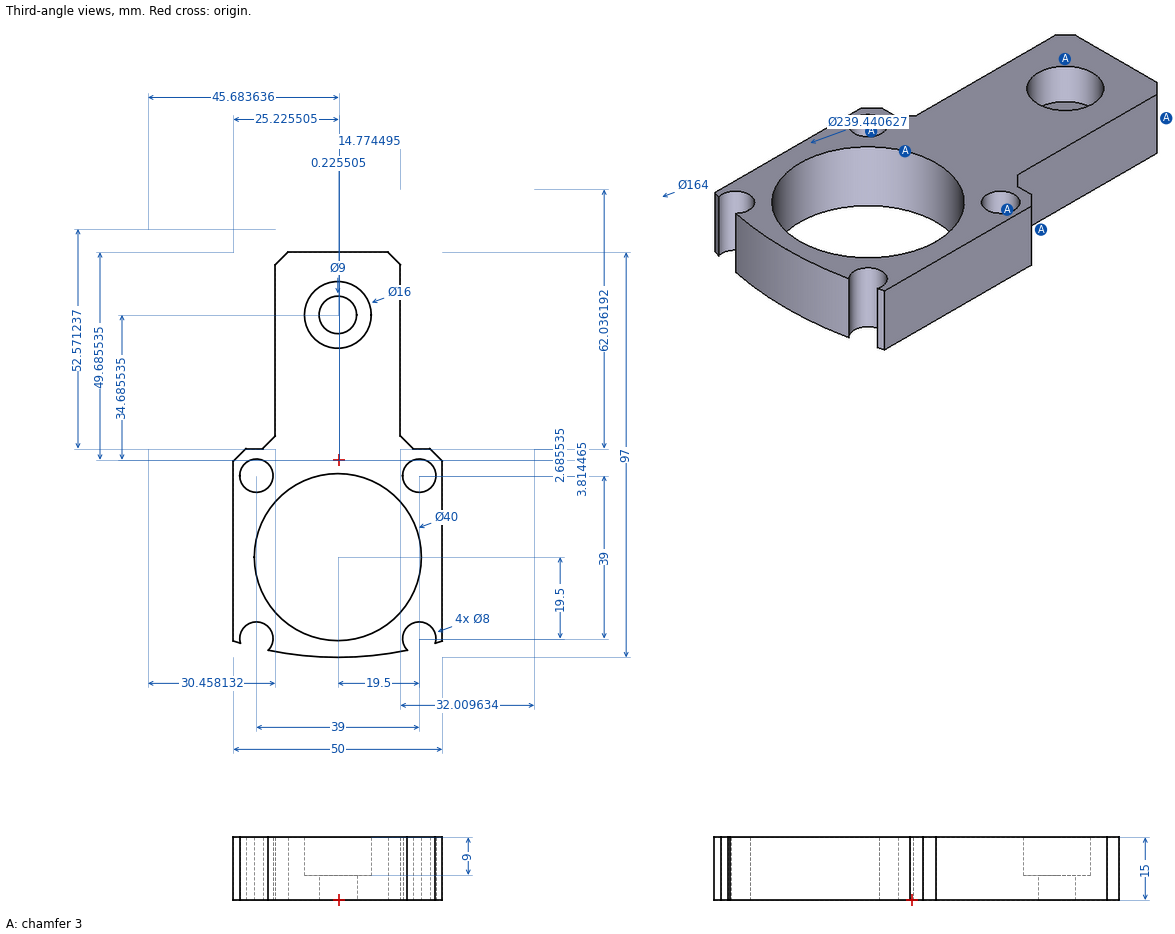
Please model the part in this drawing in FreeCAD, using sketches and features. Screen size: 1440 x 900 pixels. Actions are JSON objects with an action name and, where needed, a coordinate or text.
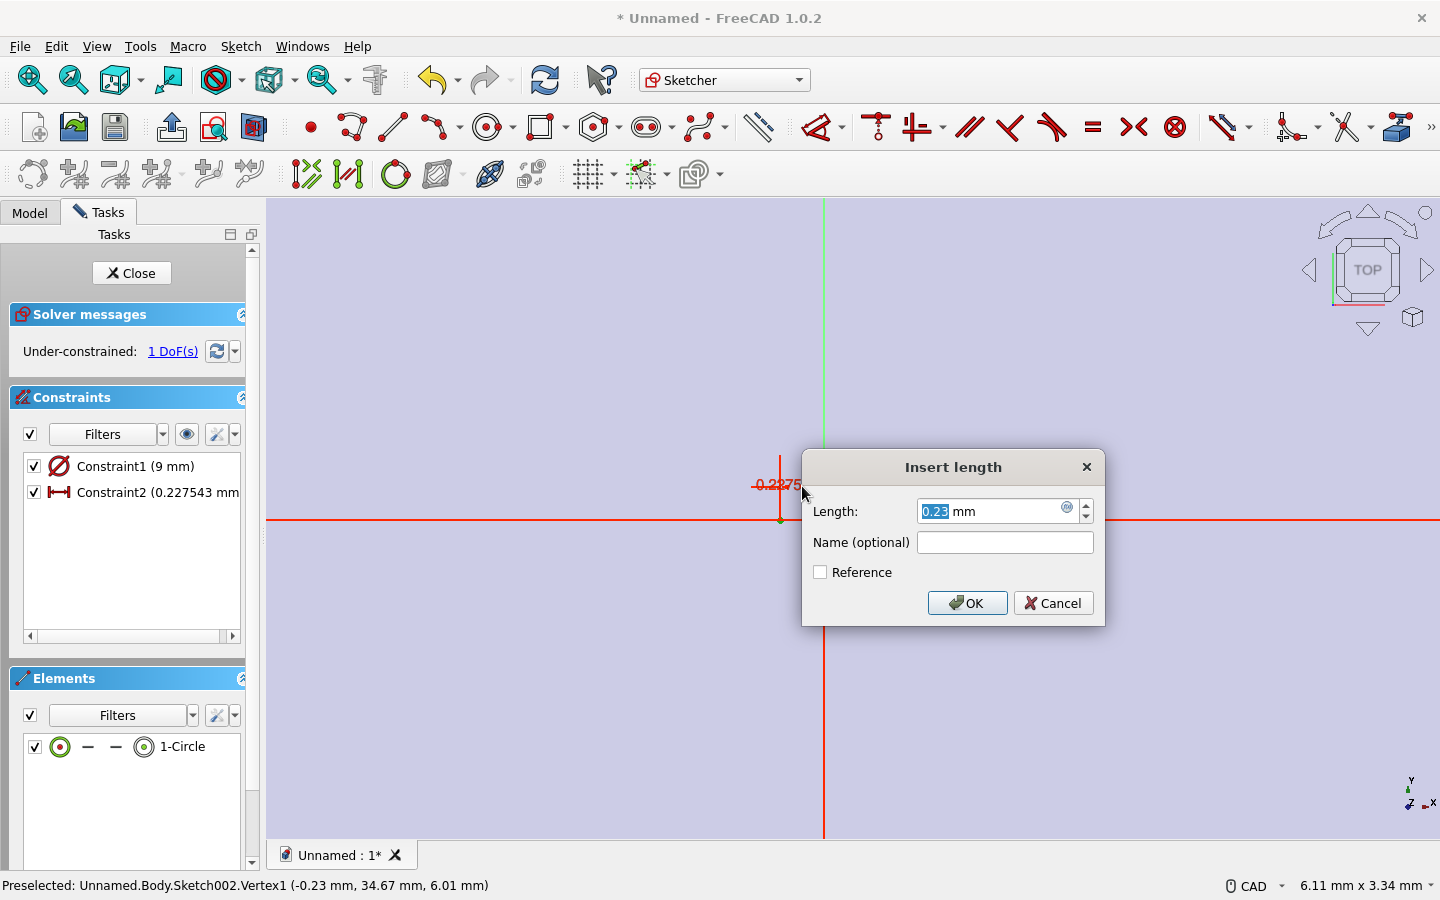
{"action": "type", "text": "0.225505"}
{"action": "key", "text": "Return"}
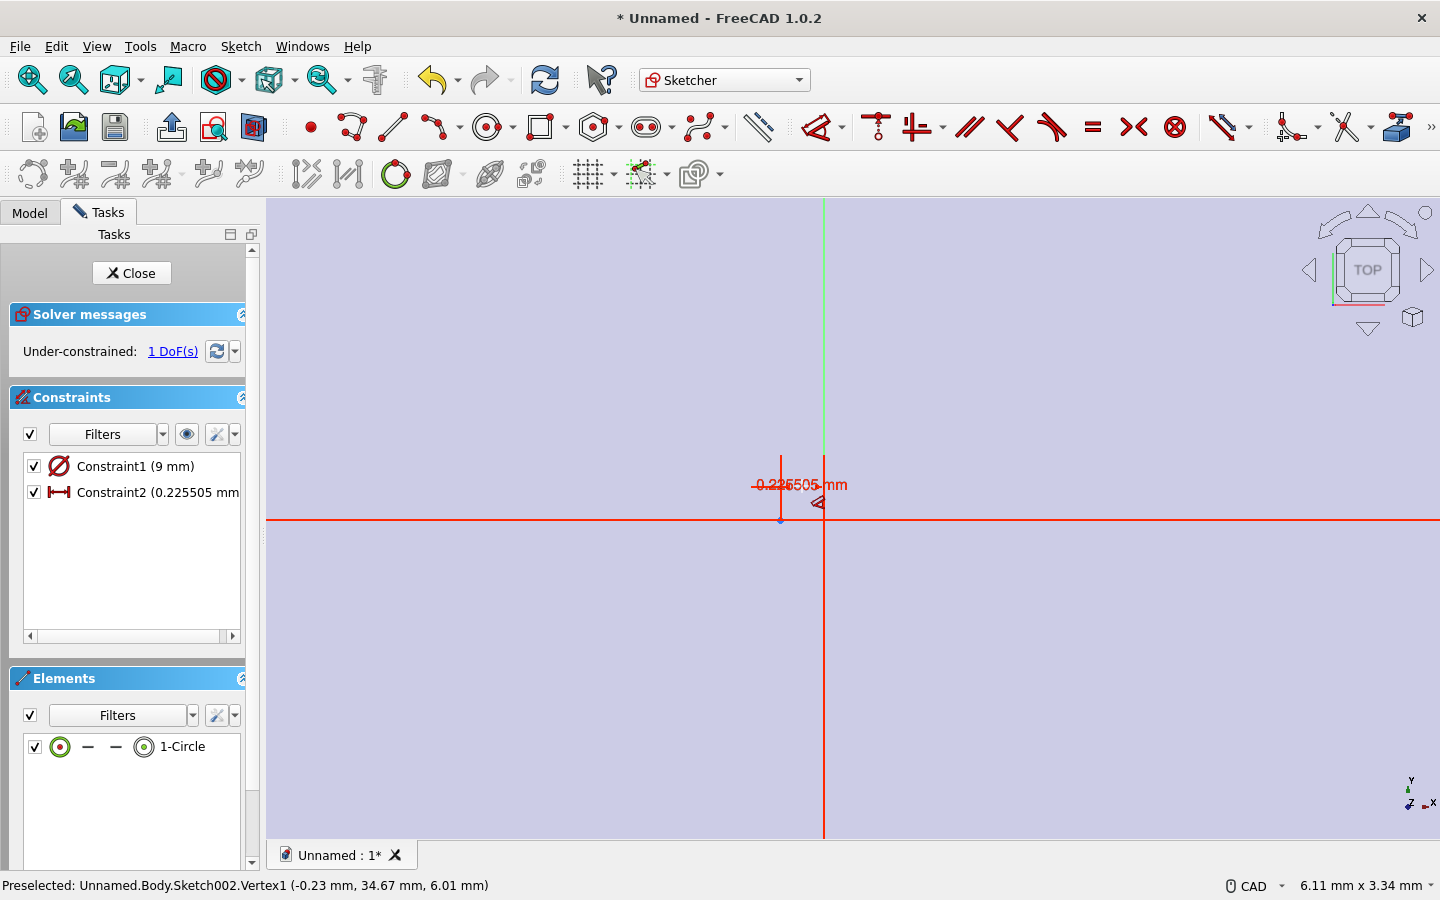
{"action": "scroll", "coordinate": [786, 519], "scroll_direction": "down", "scroll_amount": 7}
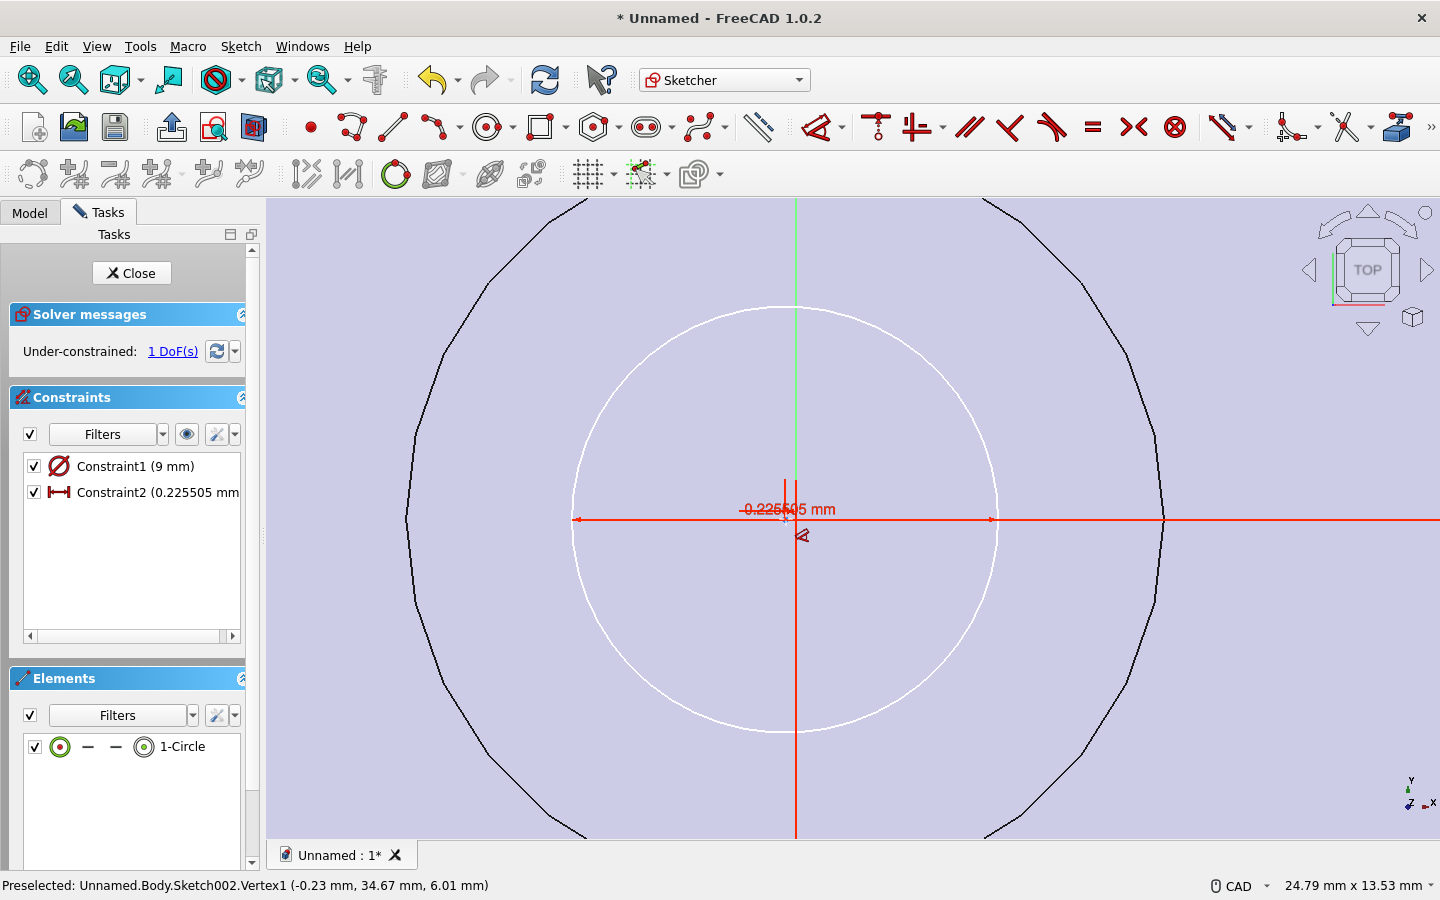
{"action": "left_click", "coordinate": [785, 520]}
{"action": "left_click", "coordinate": [830, 665]}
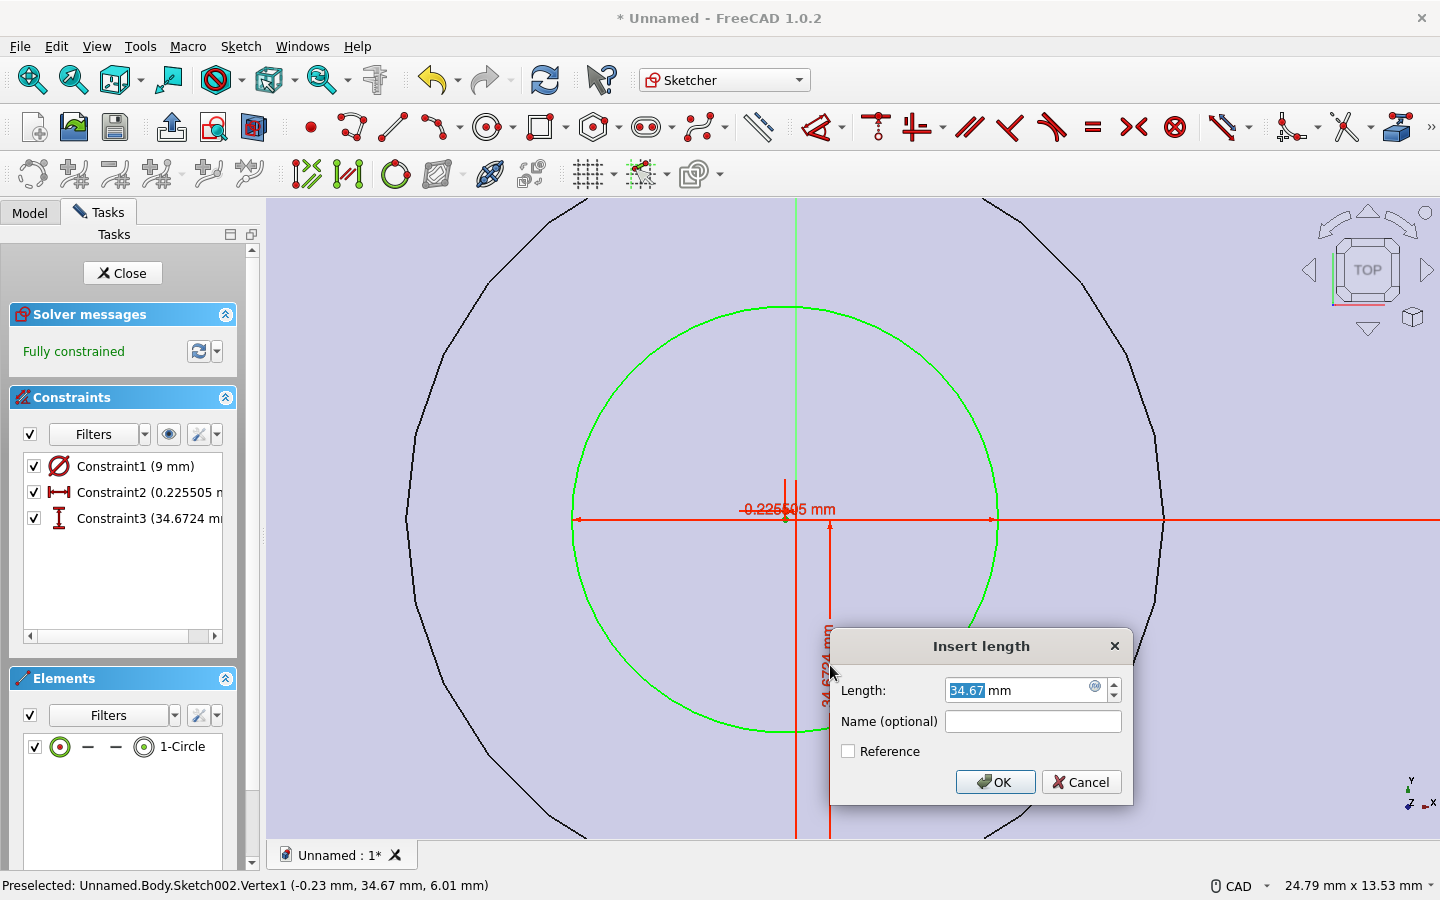
{"action": "type", "text": "34.685535"}
{"action": "key", "text": "Return"}
{"action": "key", "text": "Escape"}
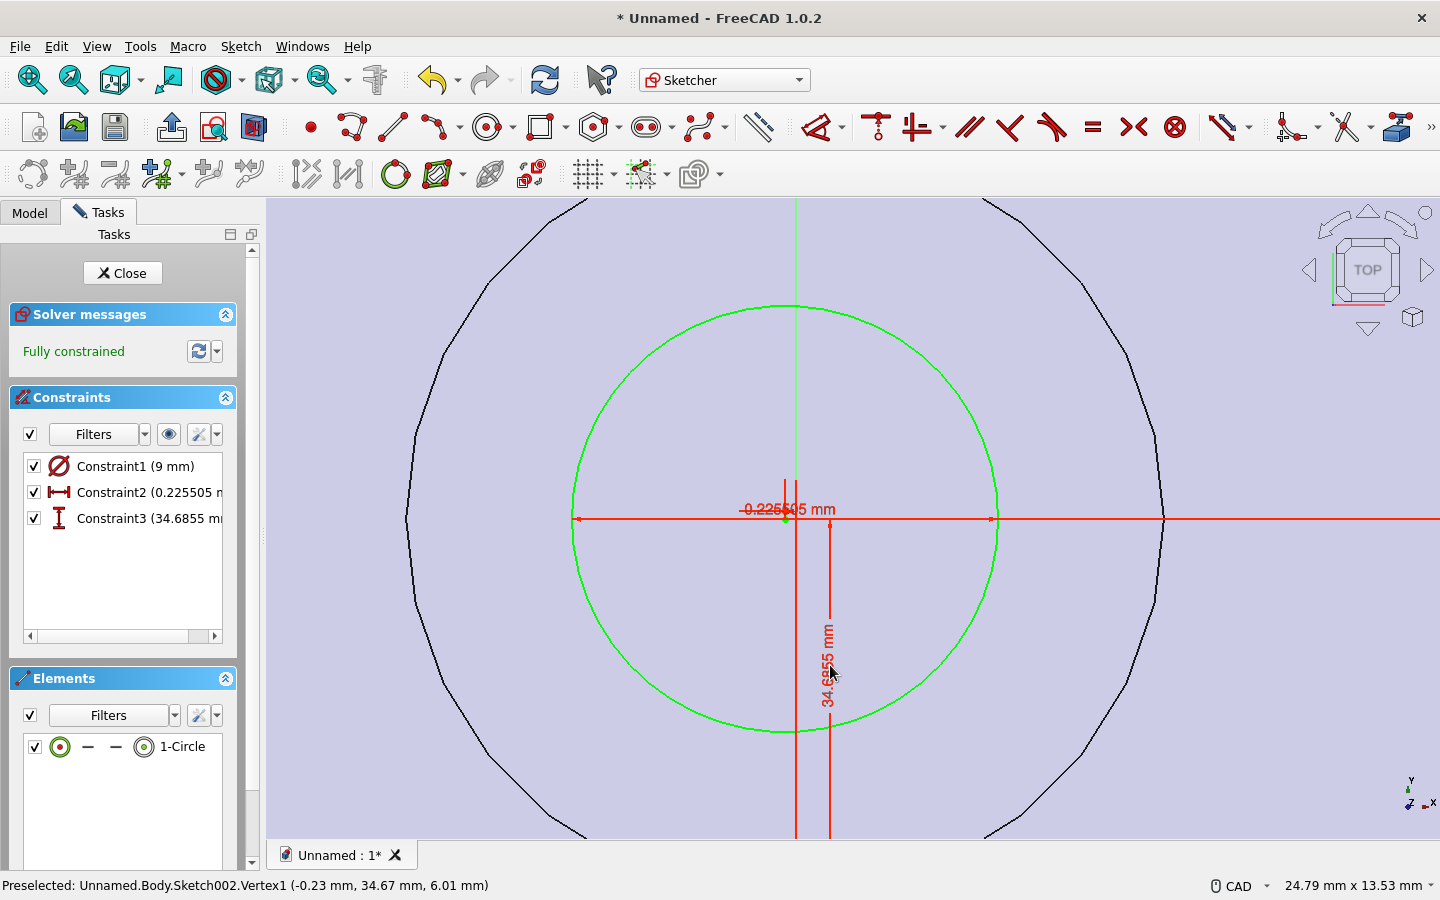
{"action": "left_click", "coordinate": [123, 273]}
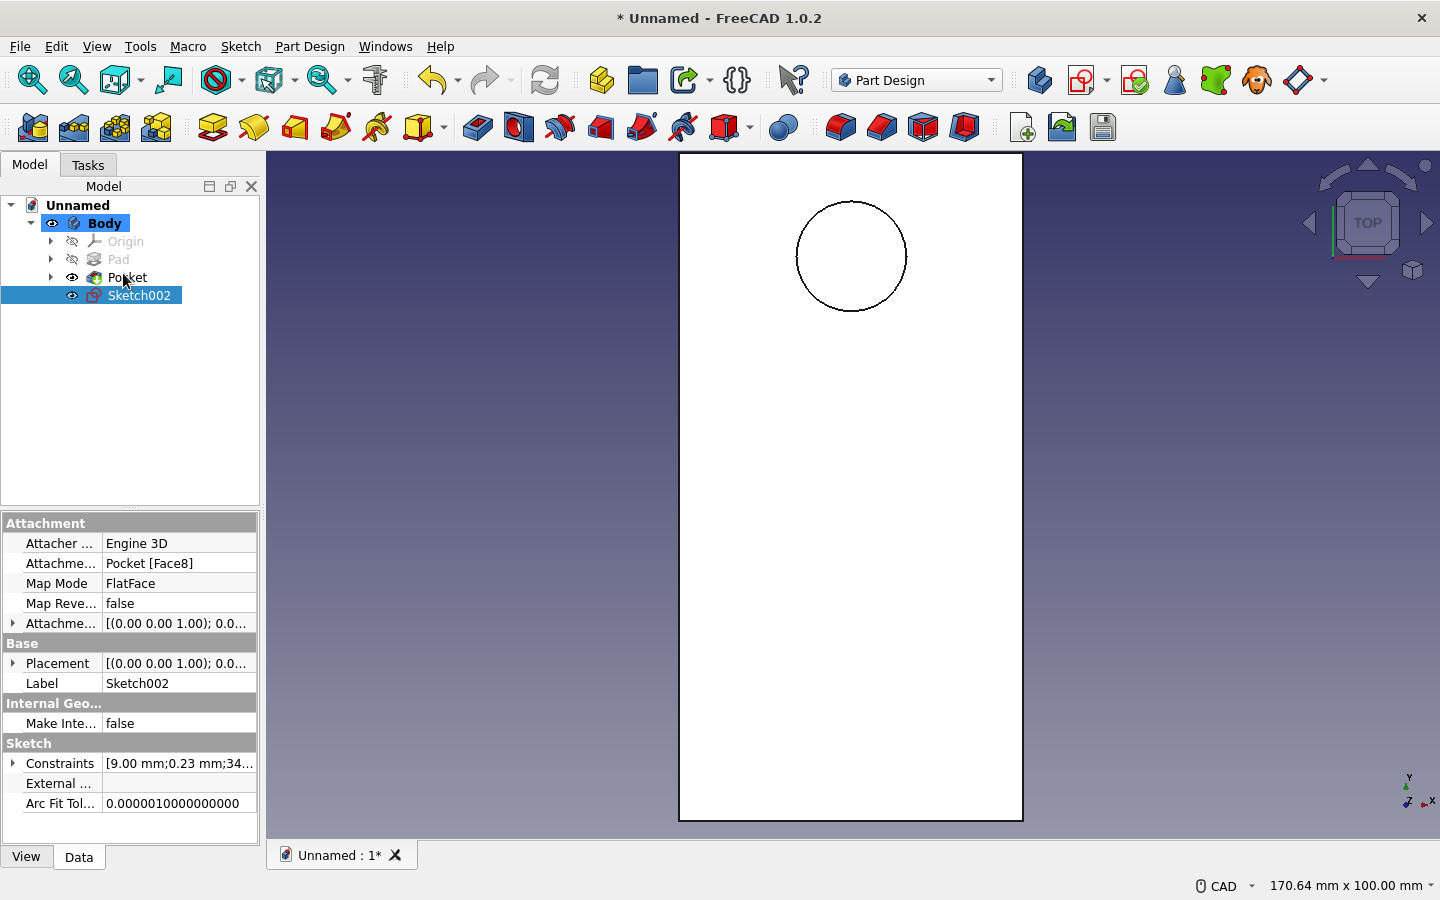
{"action": "left_click", "coordinate": [478, 128]}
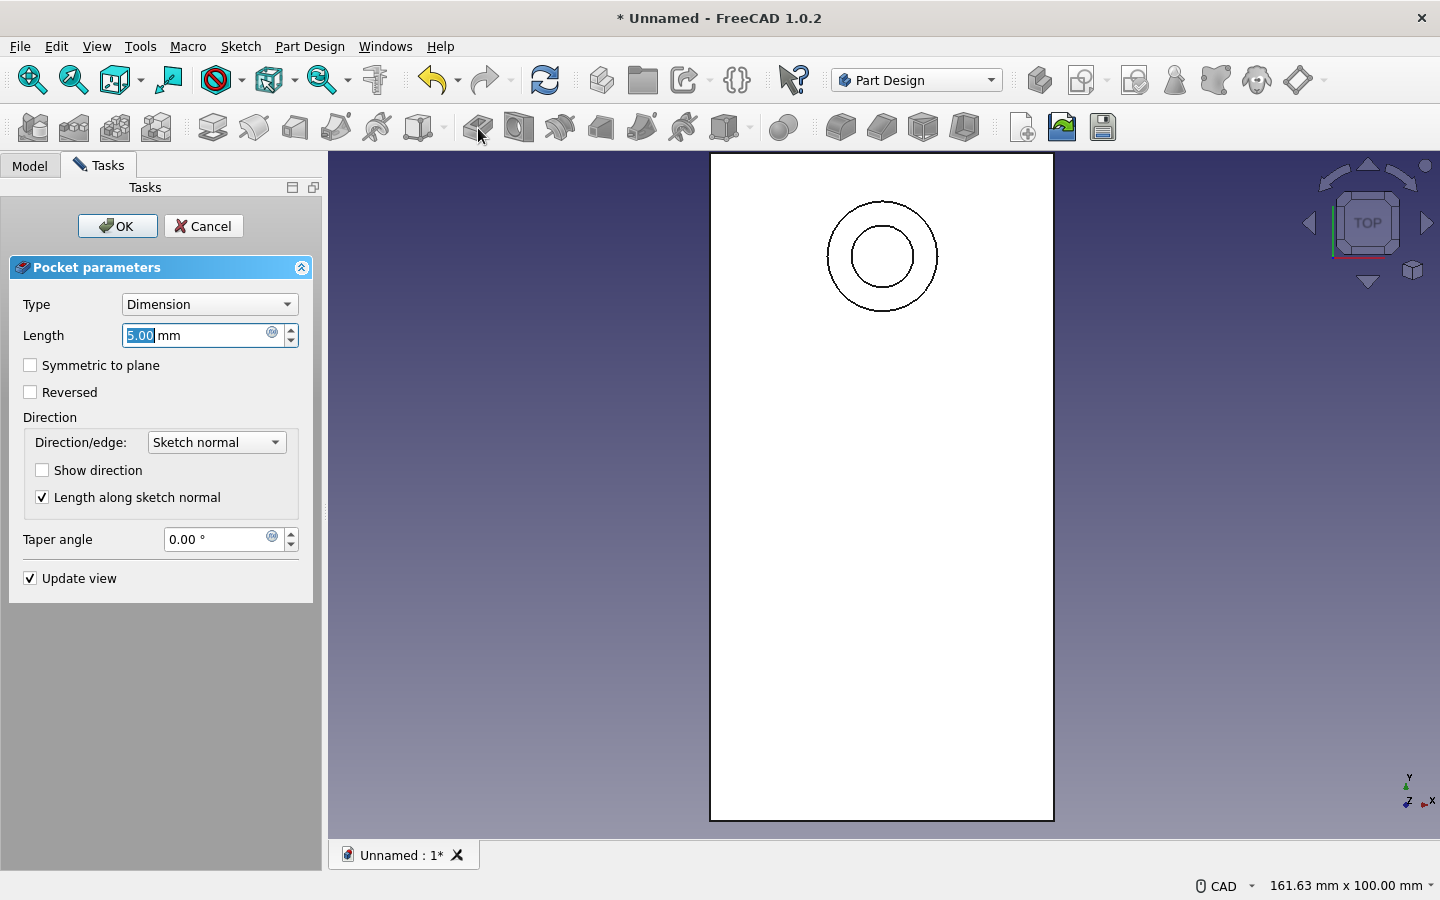
{"action": "left_click", "coordinate": [210, 304]}